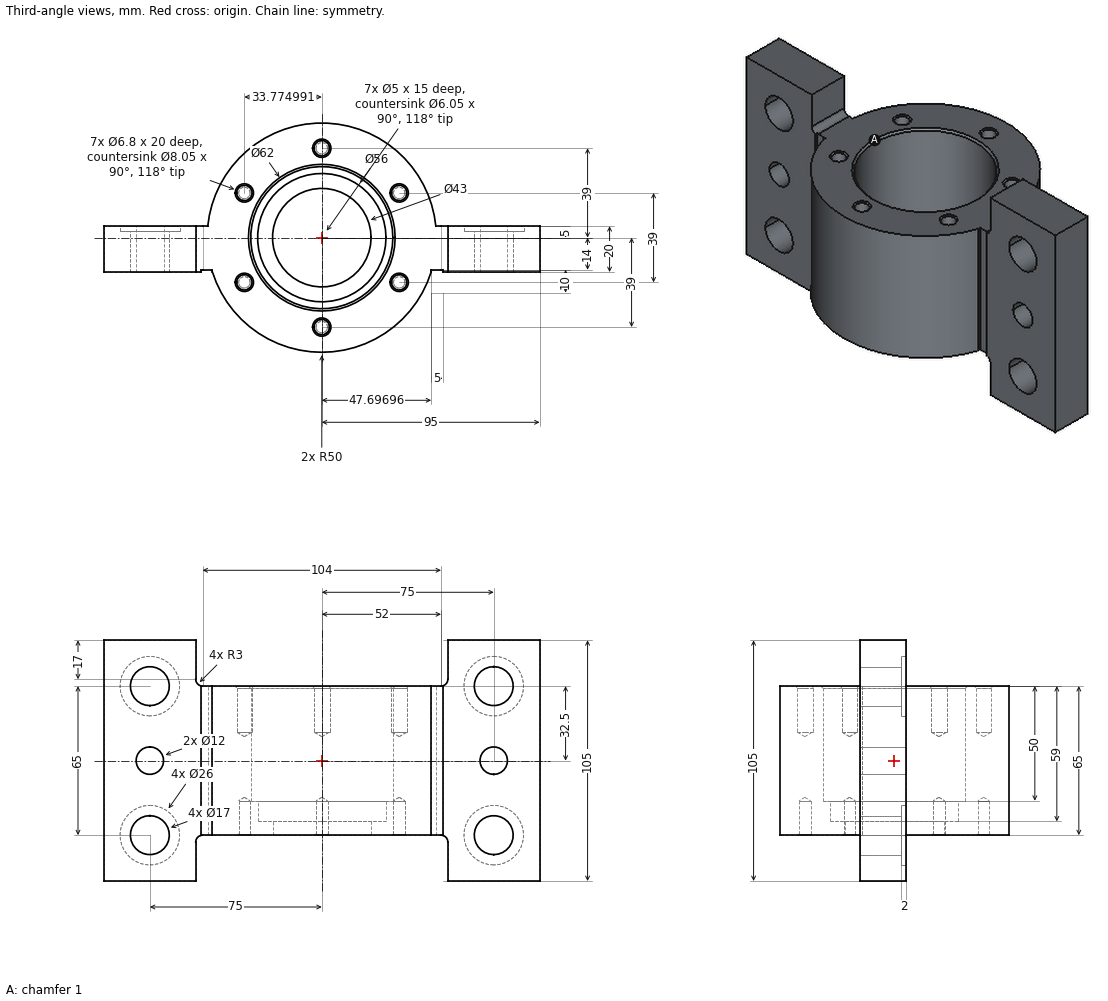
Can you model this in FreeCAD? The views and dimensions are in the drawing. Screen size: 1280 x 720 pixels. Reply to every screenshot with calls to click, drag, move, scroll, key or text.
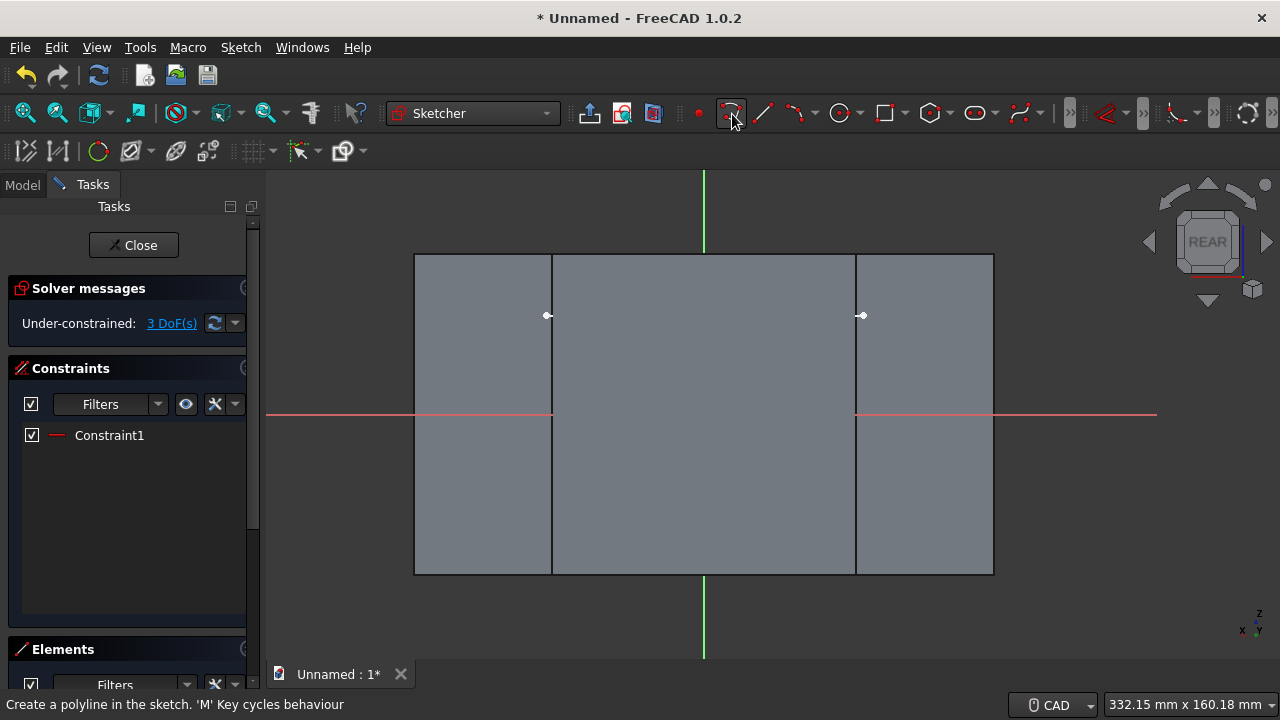
scroll(872, 306, up, 2)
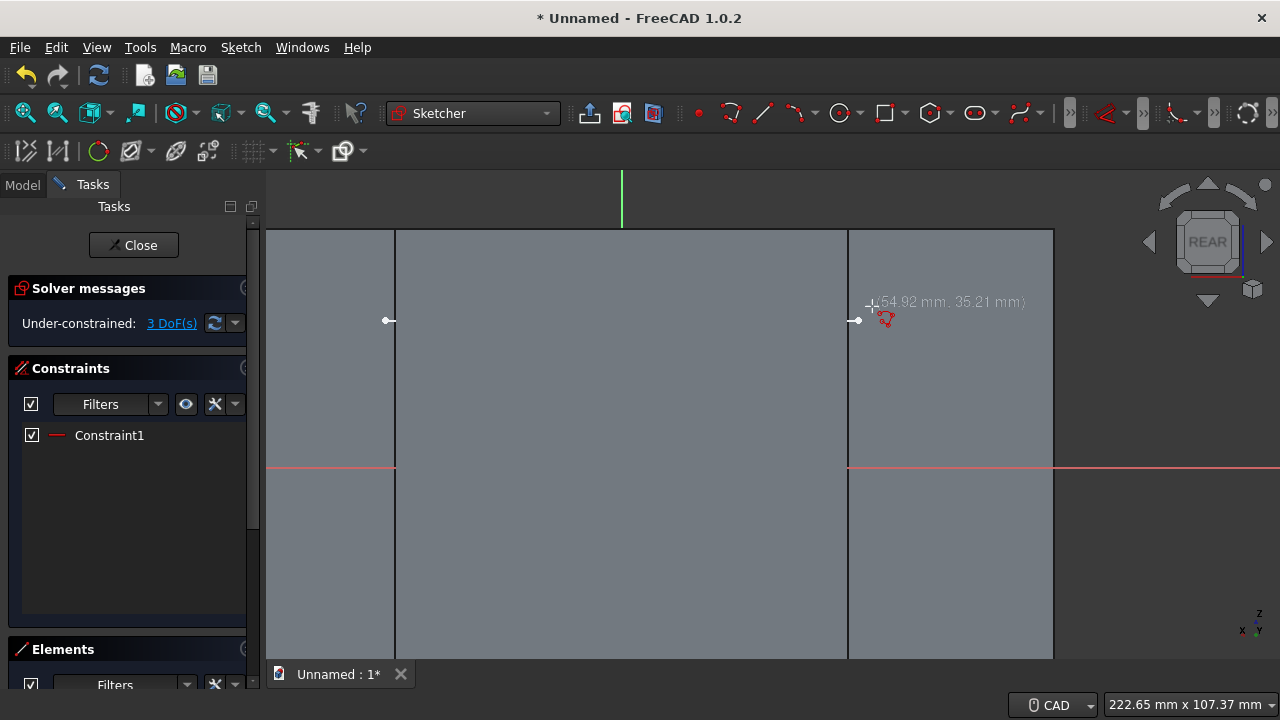
click(872, 306)
click(872, 229)
click(371, 229)
click(371, 306)
right_click(371, 306)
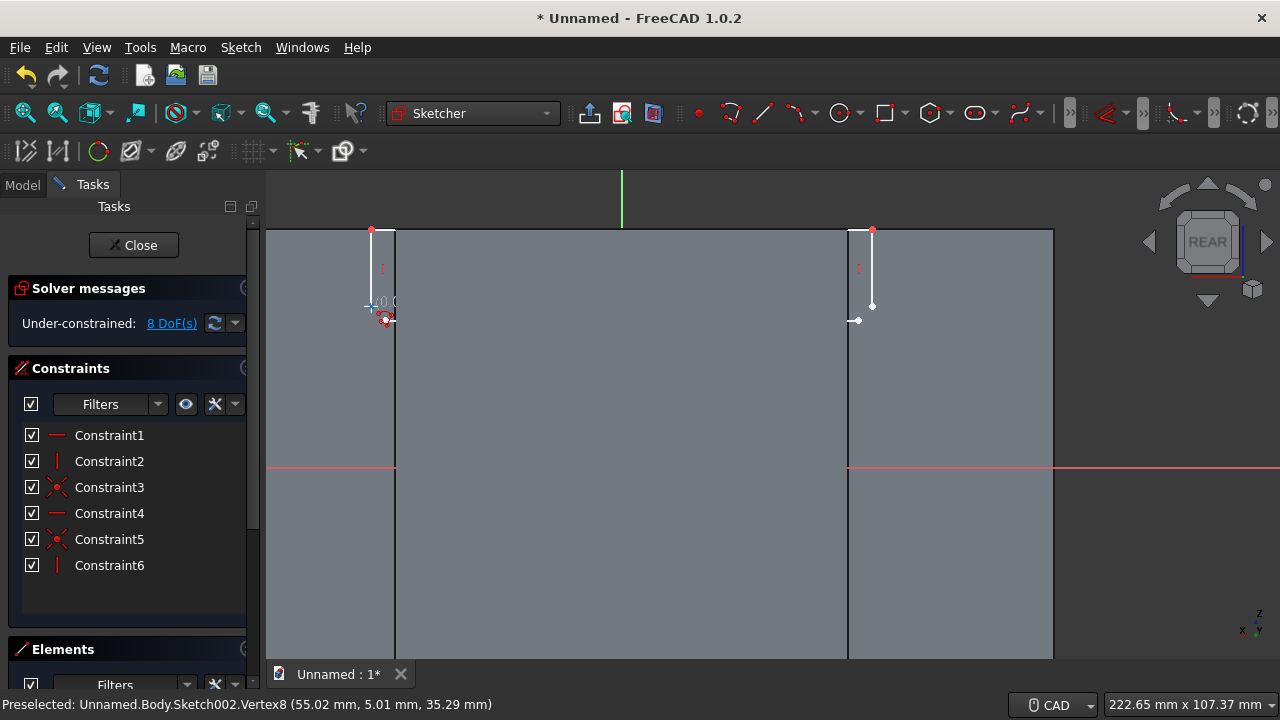
click(796, 114)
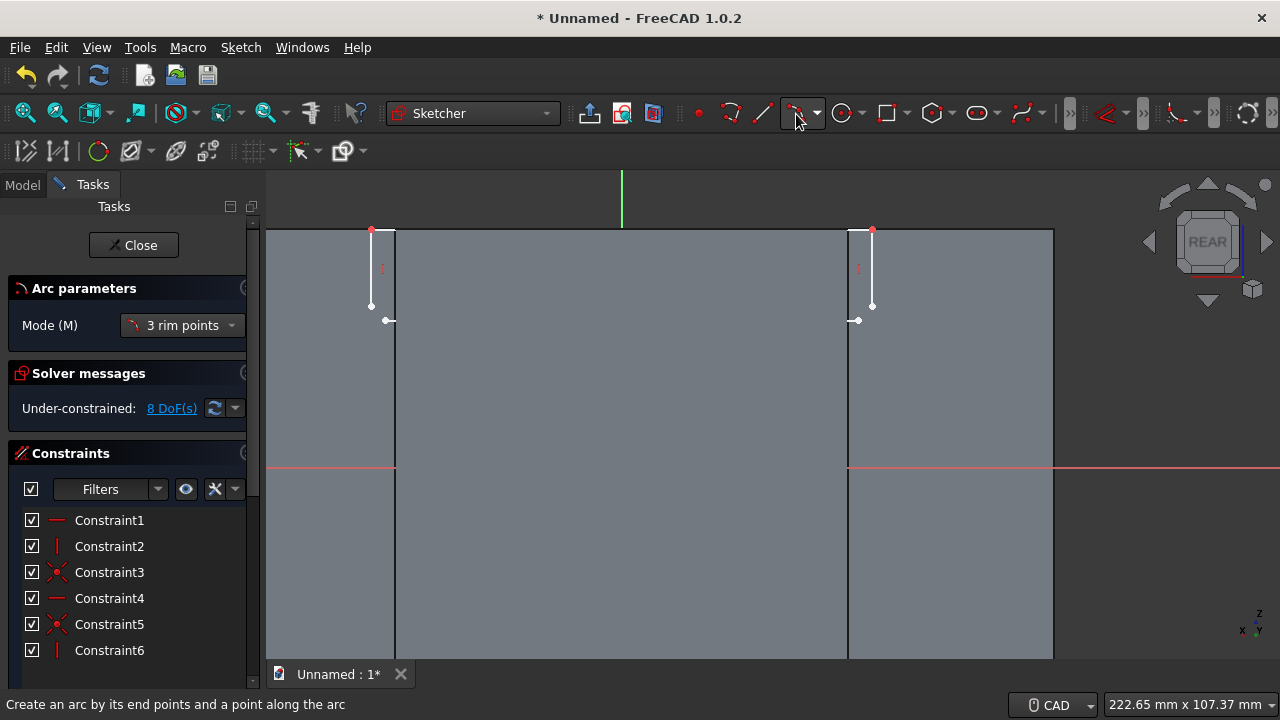
click(858, 321)
click(872, 307)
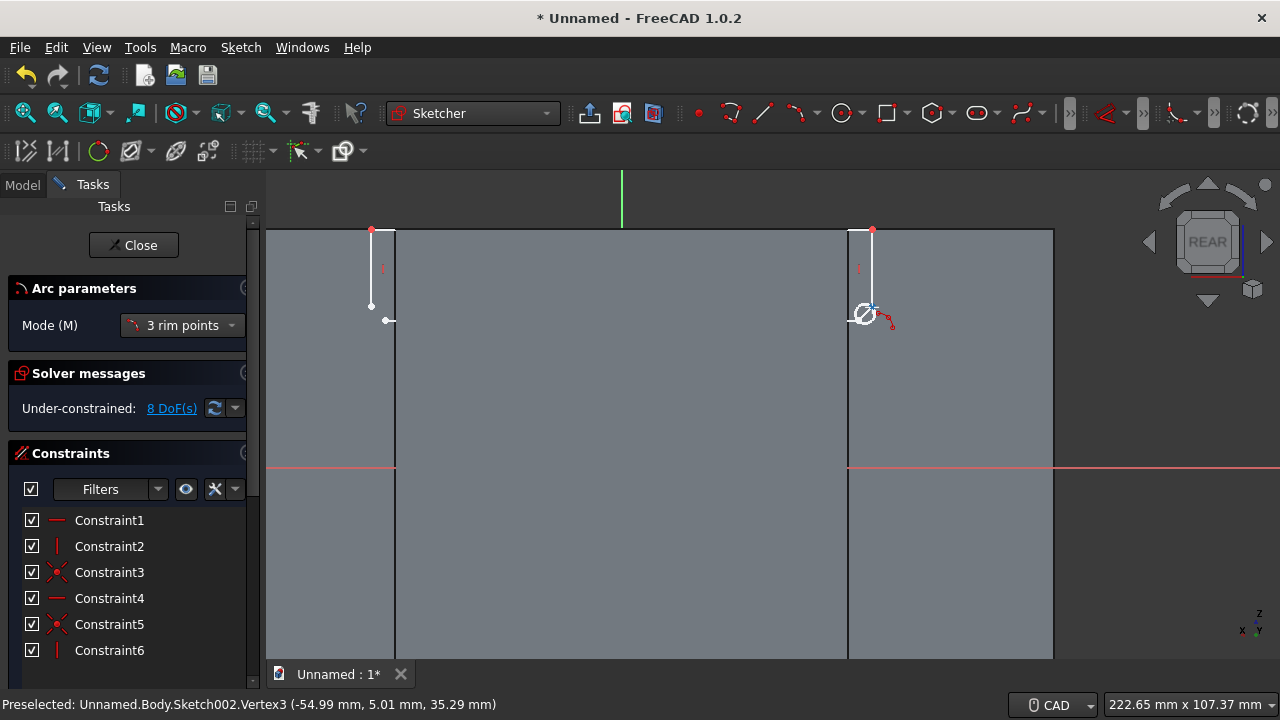
scroll(868, 316, up, 7)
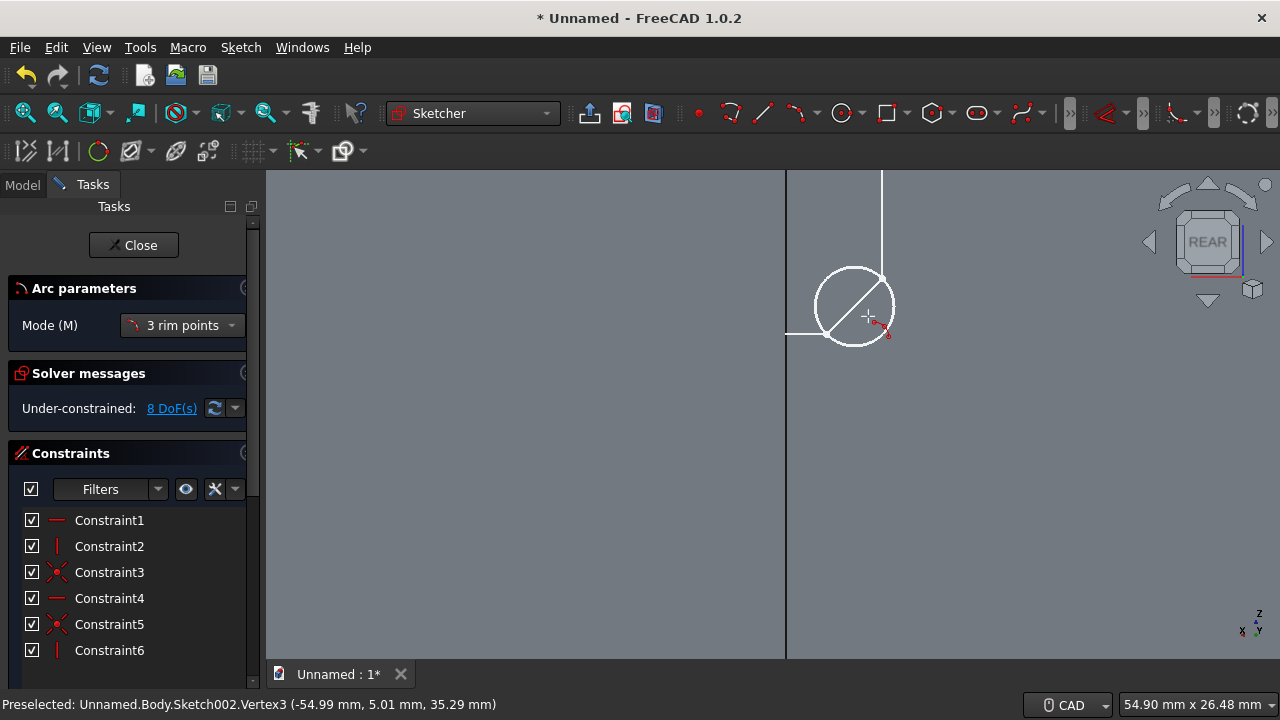
click(866, 314)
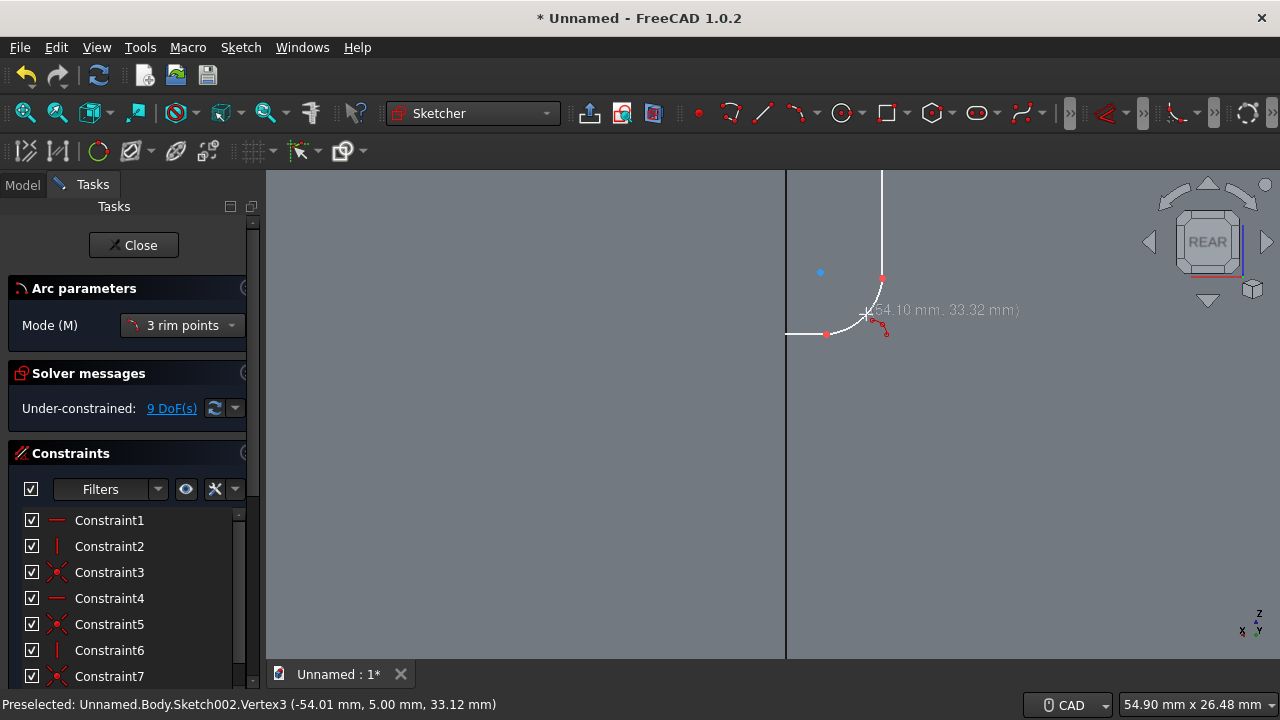
scroll(870, 312, down, 9)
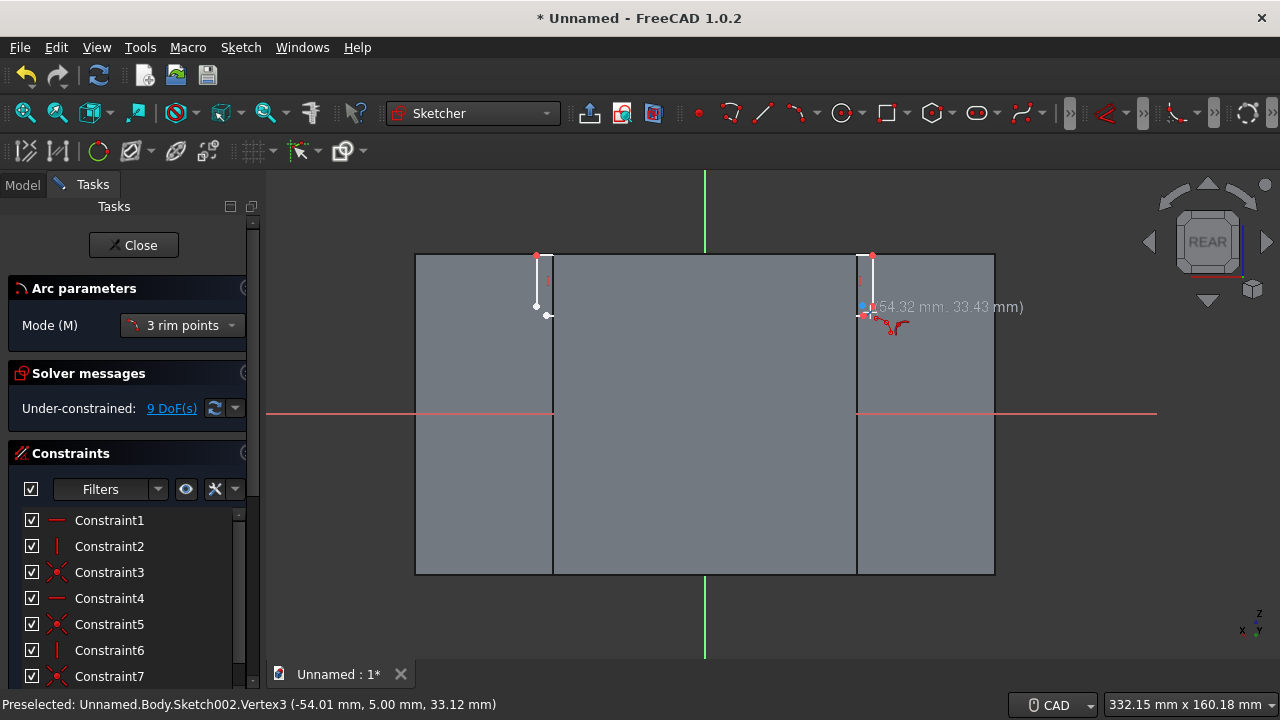
scroll(537, 306, up, 2)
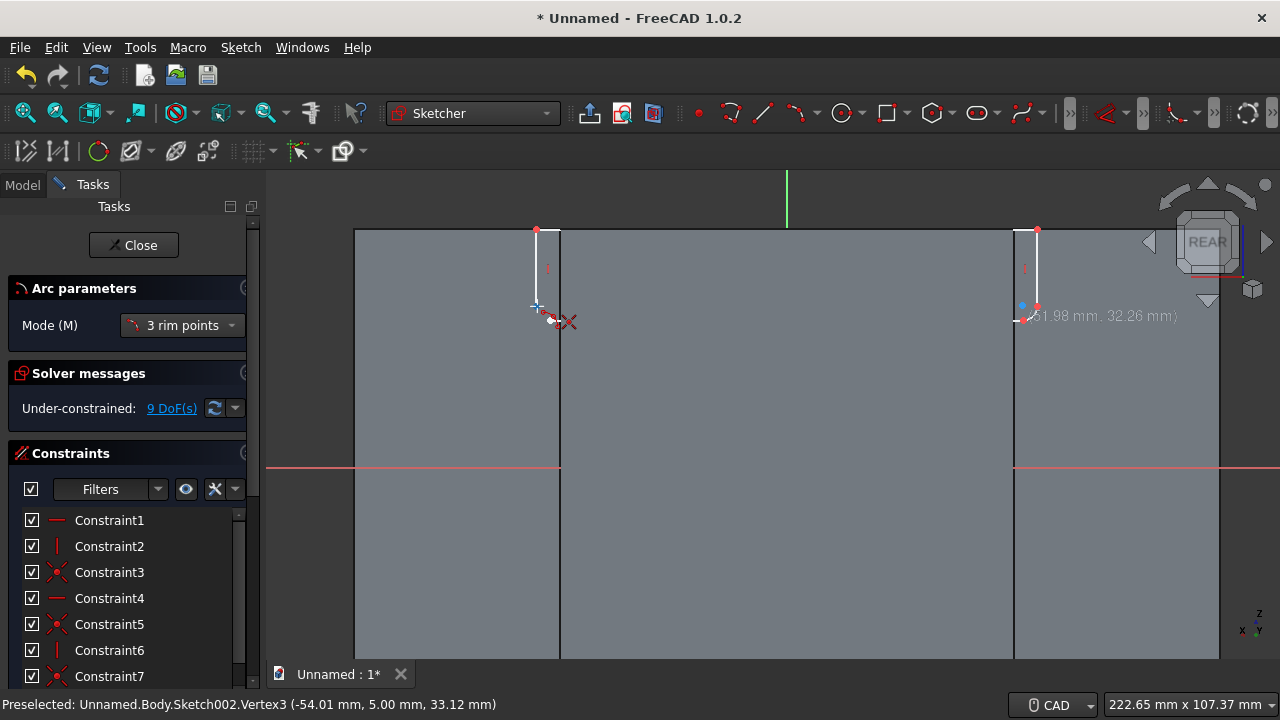
click(536, 307)
click(551, 321)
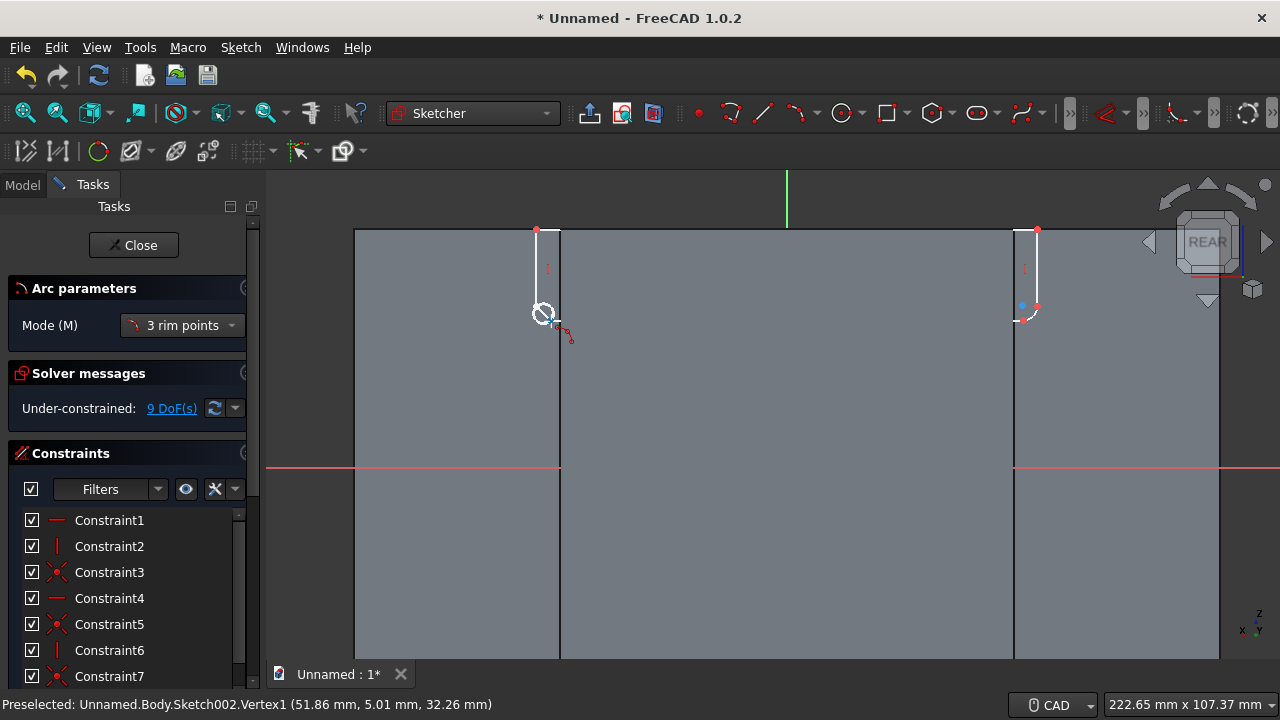
scroll(541, 316, up, 7)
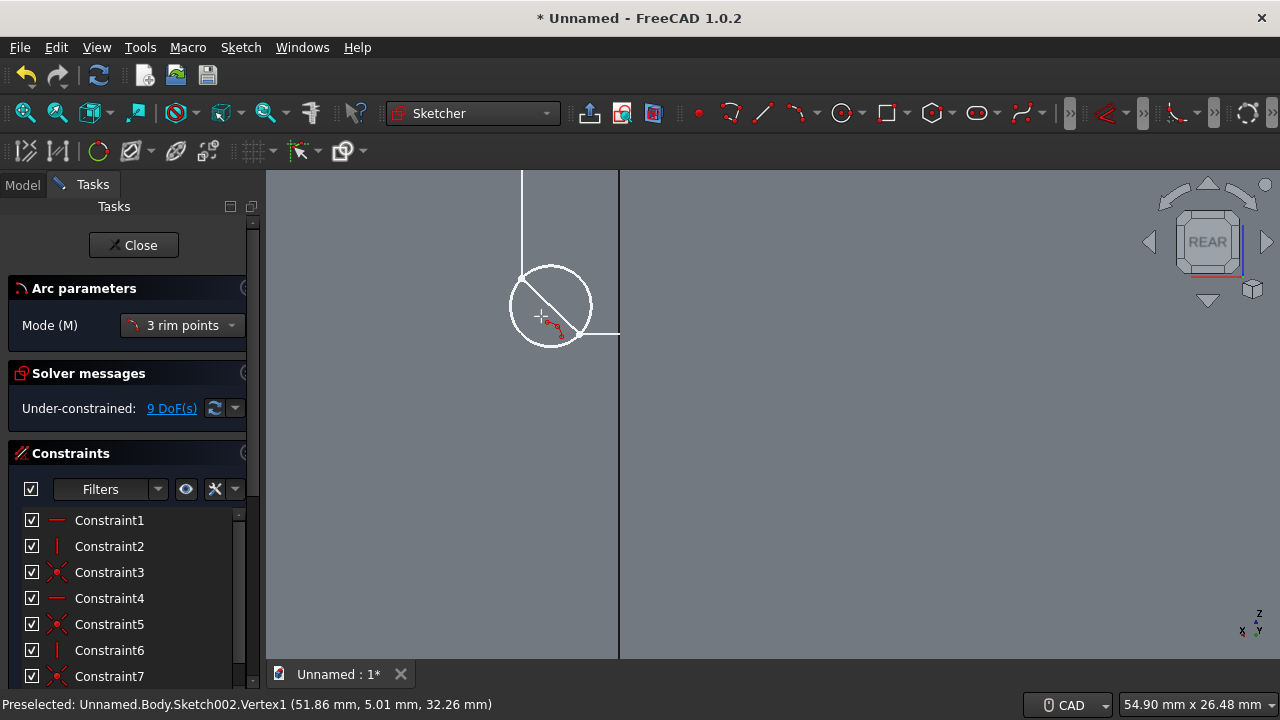
click(538, 314)